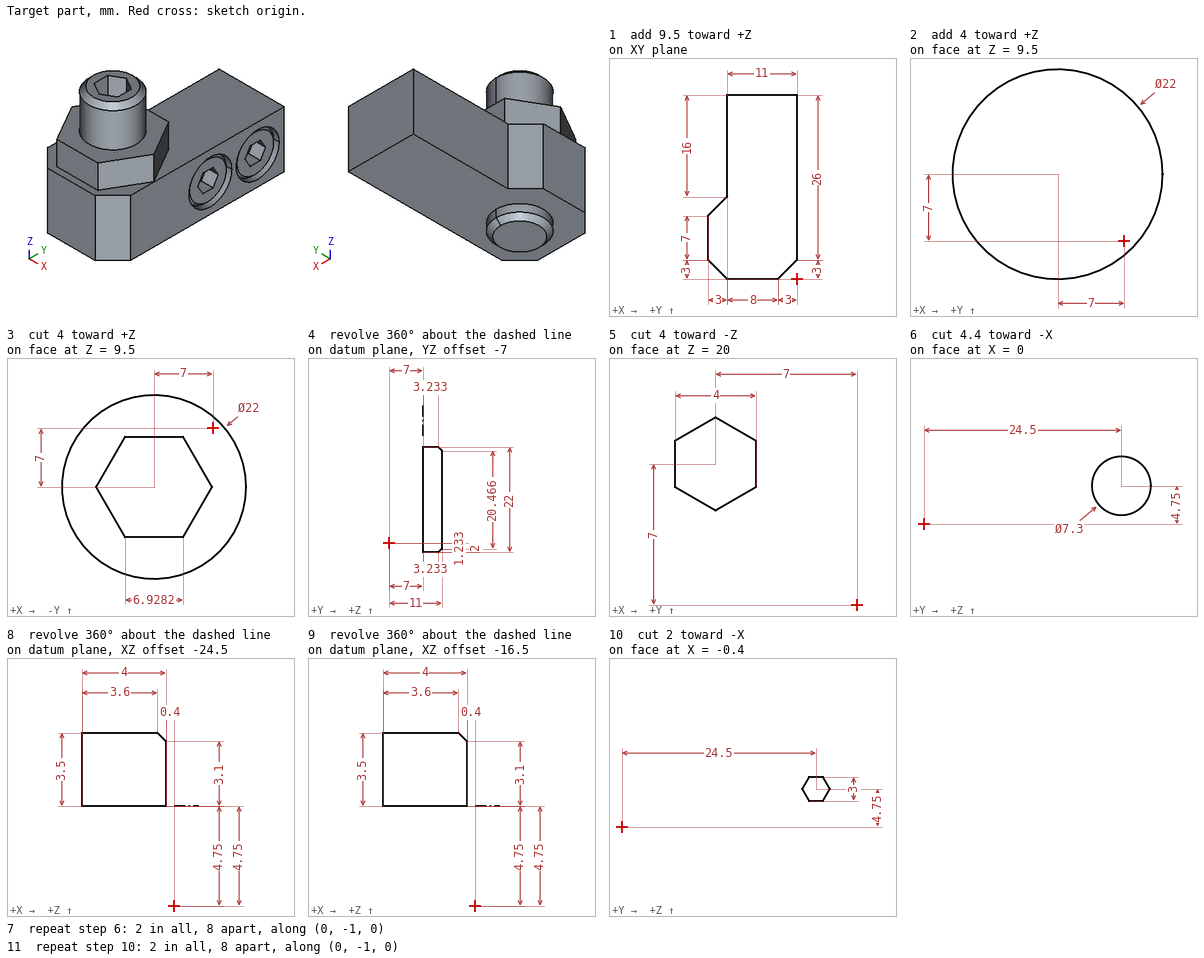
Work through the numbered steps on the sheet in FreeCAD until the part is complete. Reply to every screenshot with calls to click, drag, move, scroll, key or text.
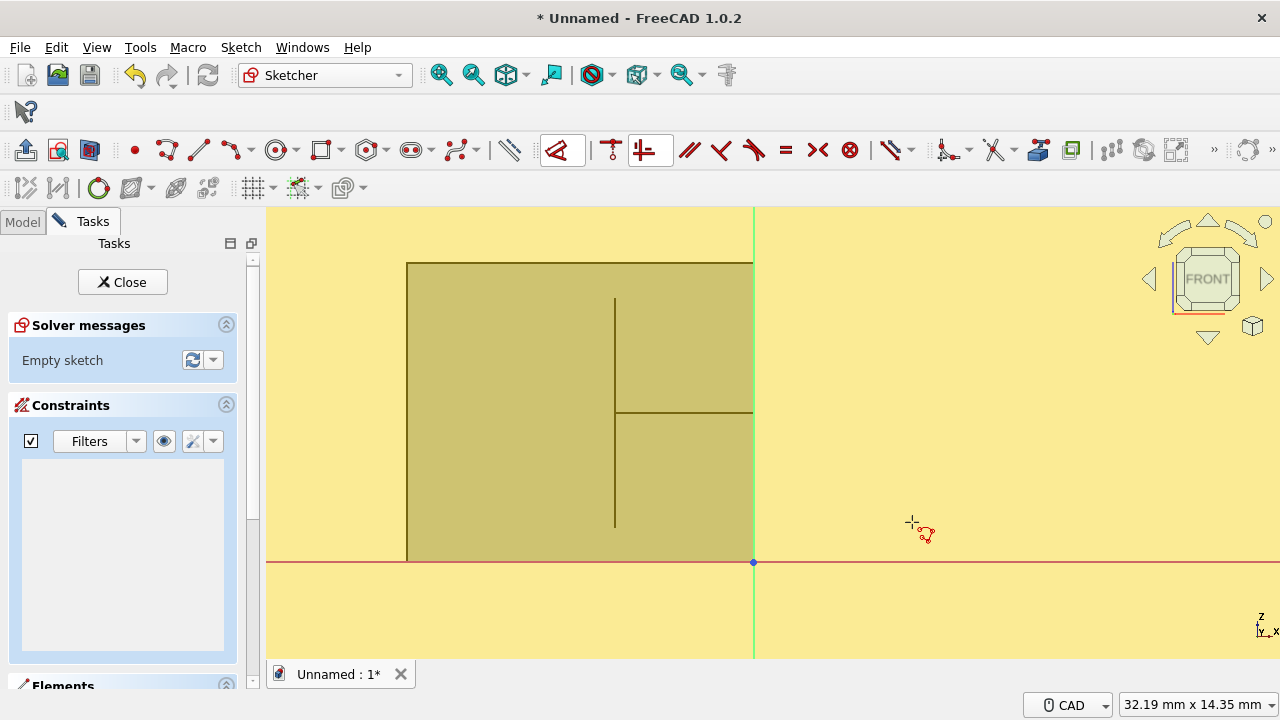
scroll(741, 413, up, 2)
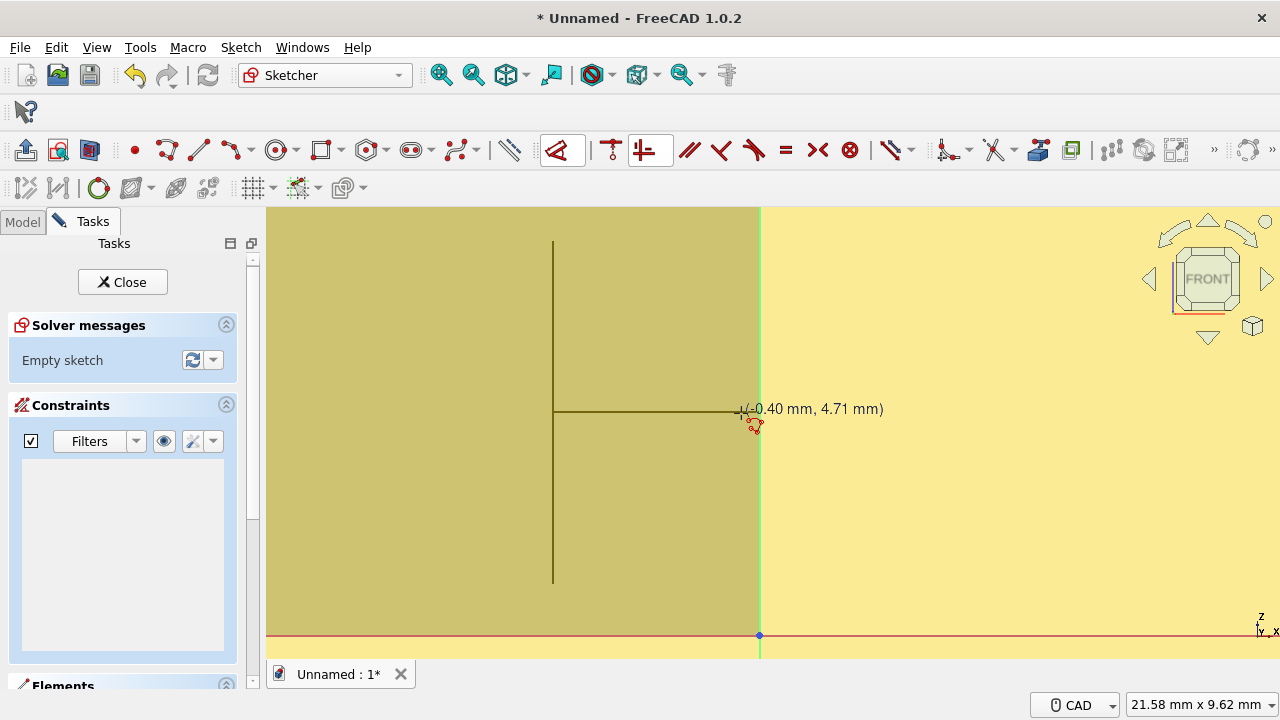
click(741, 412)
click(553, 412)
click(553, 248)
click(722, 248)
click(741, 267)
click(741, 413)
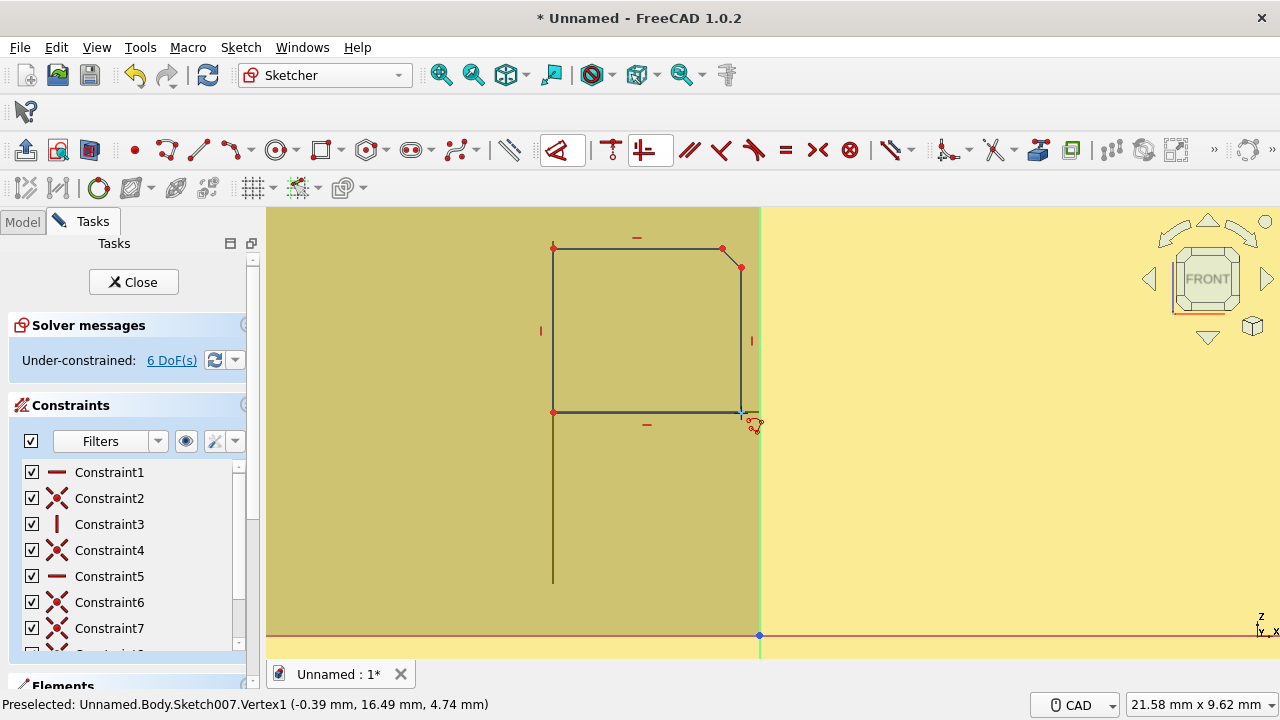
click(200, 150)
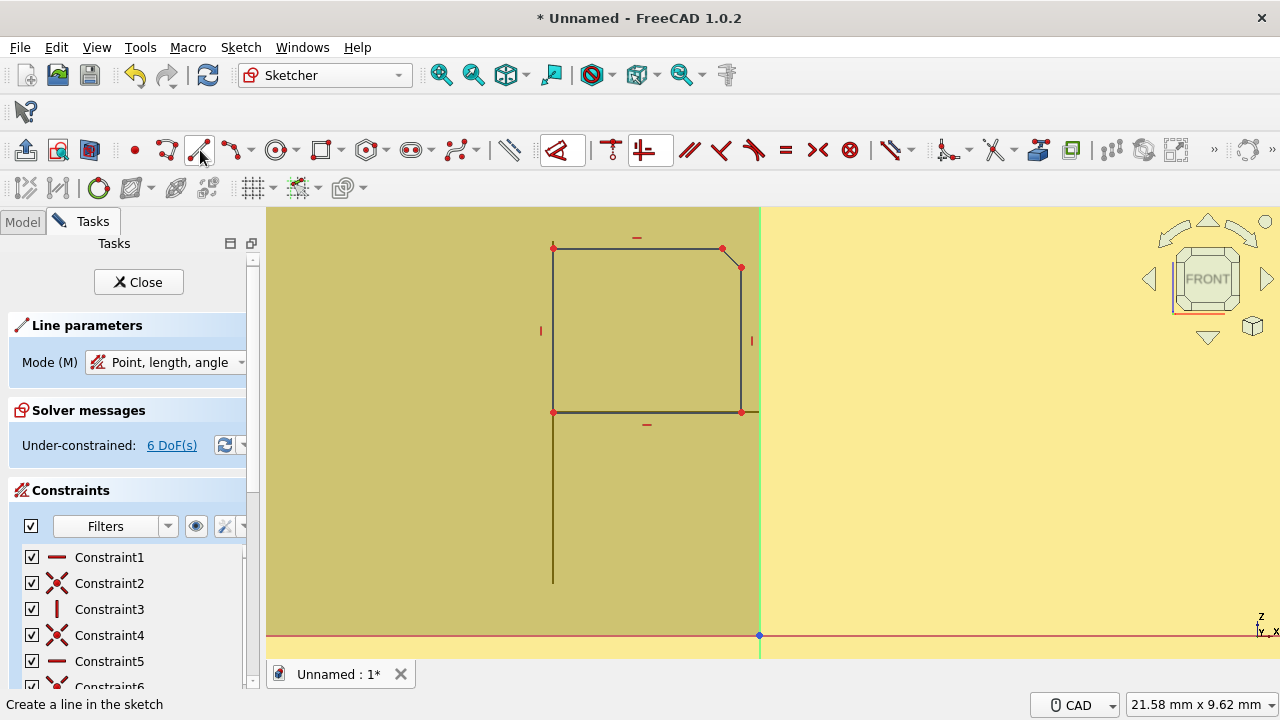
click(760, 412)
click(816, 412)
key(Escape)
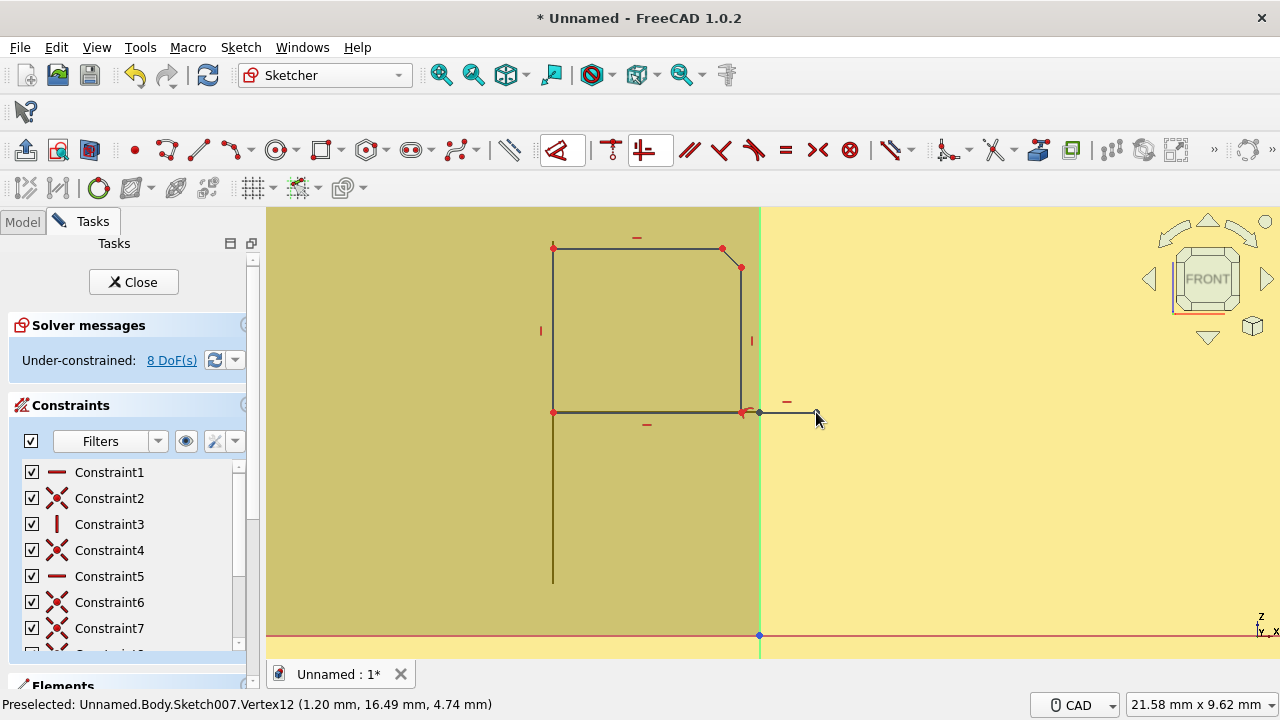
click(776, 413)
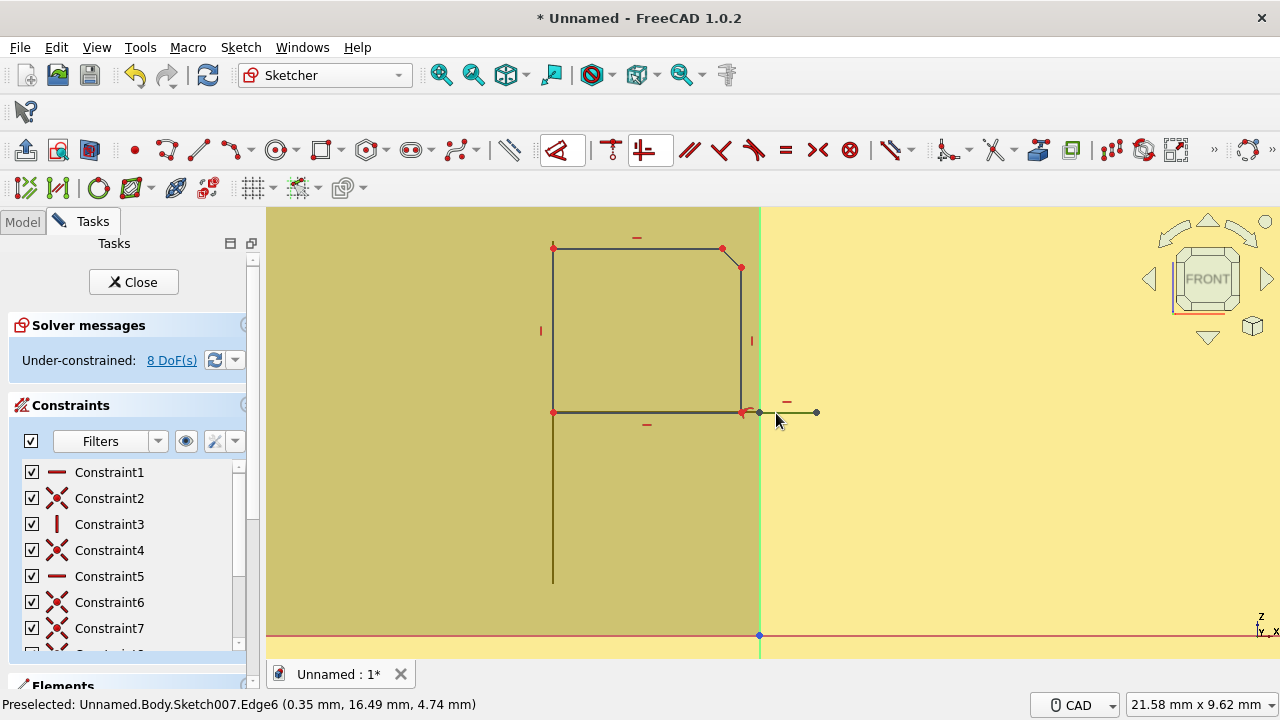
key(g)
key(n)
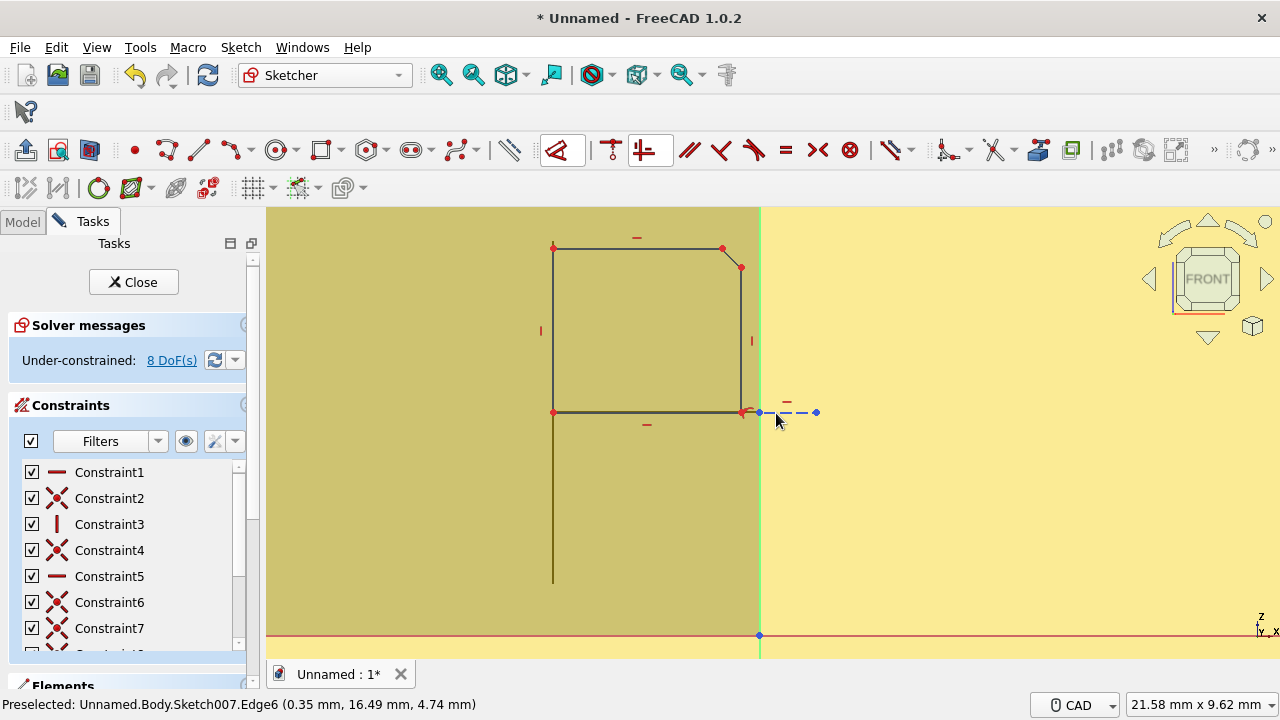
click(685, 413)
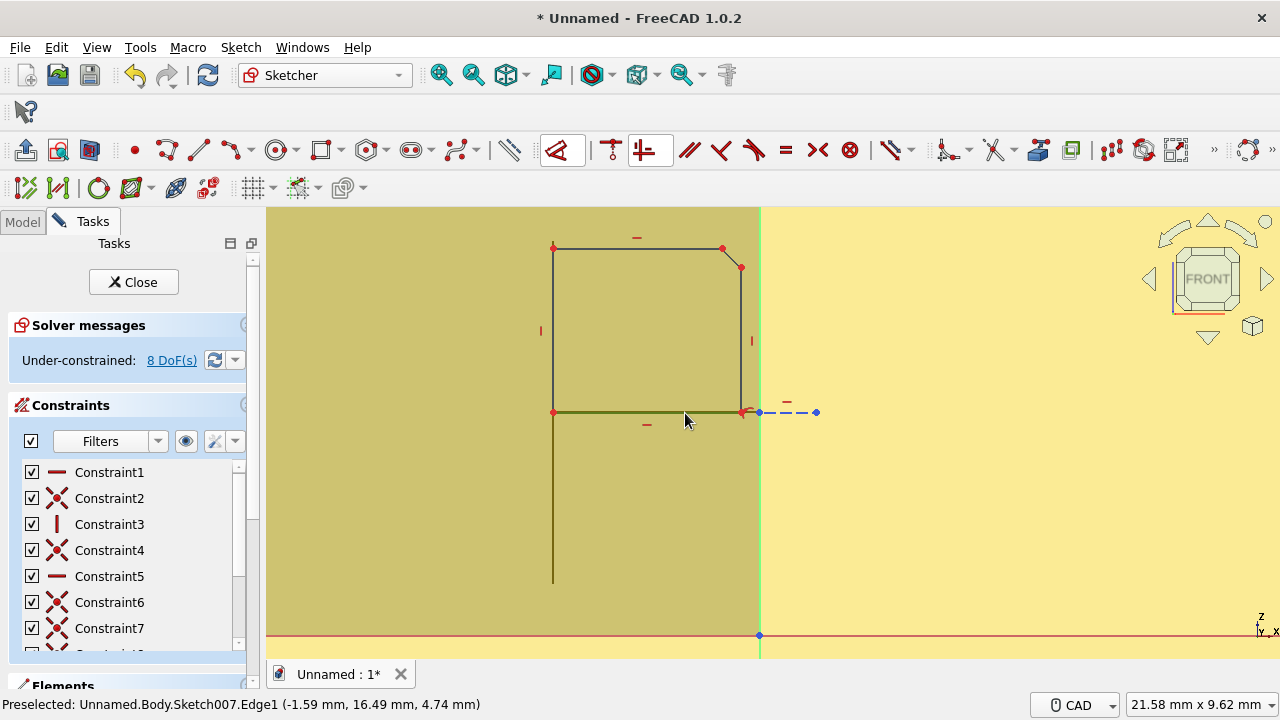
key(l)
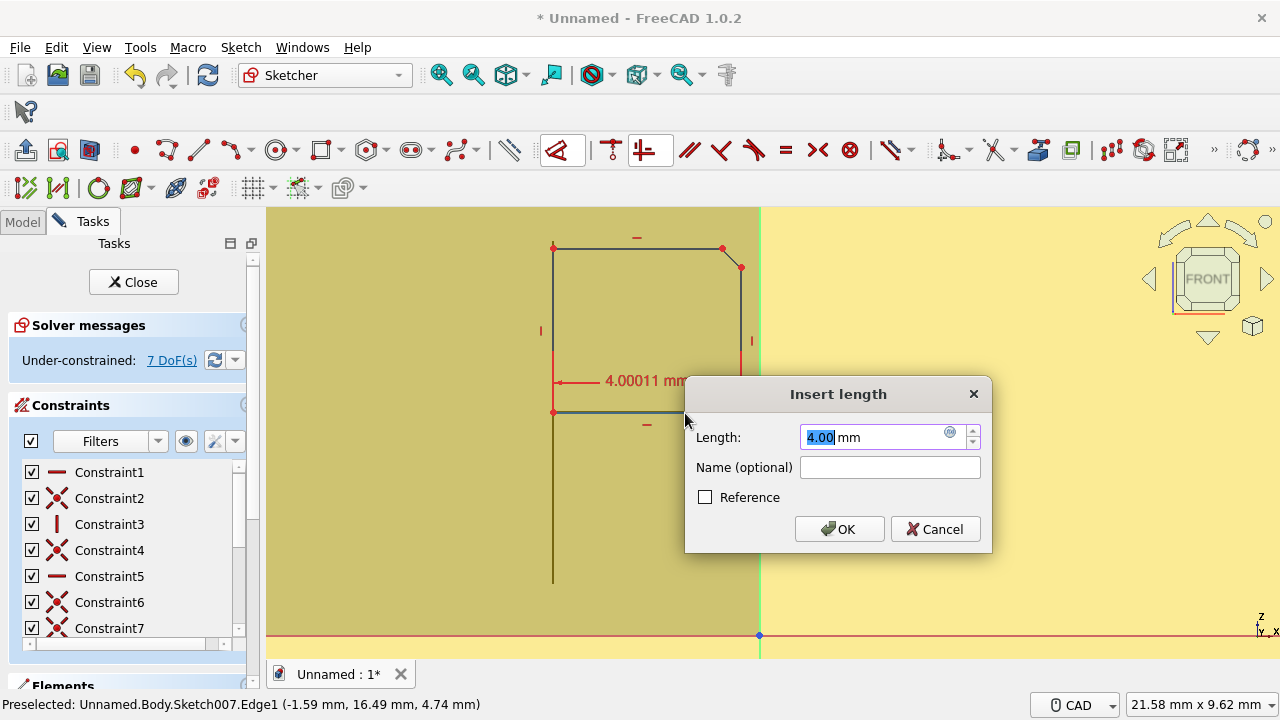
text(4)
key(Return)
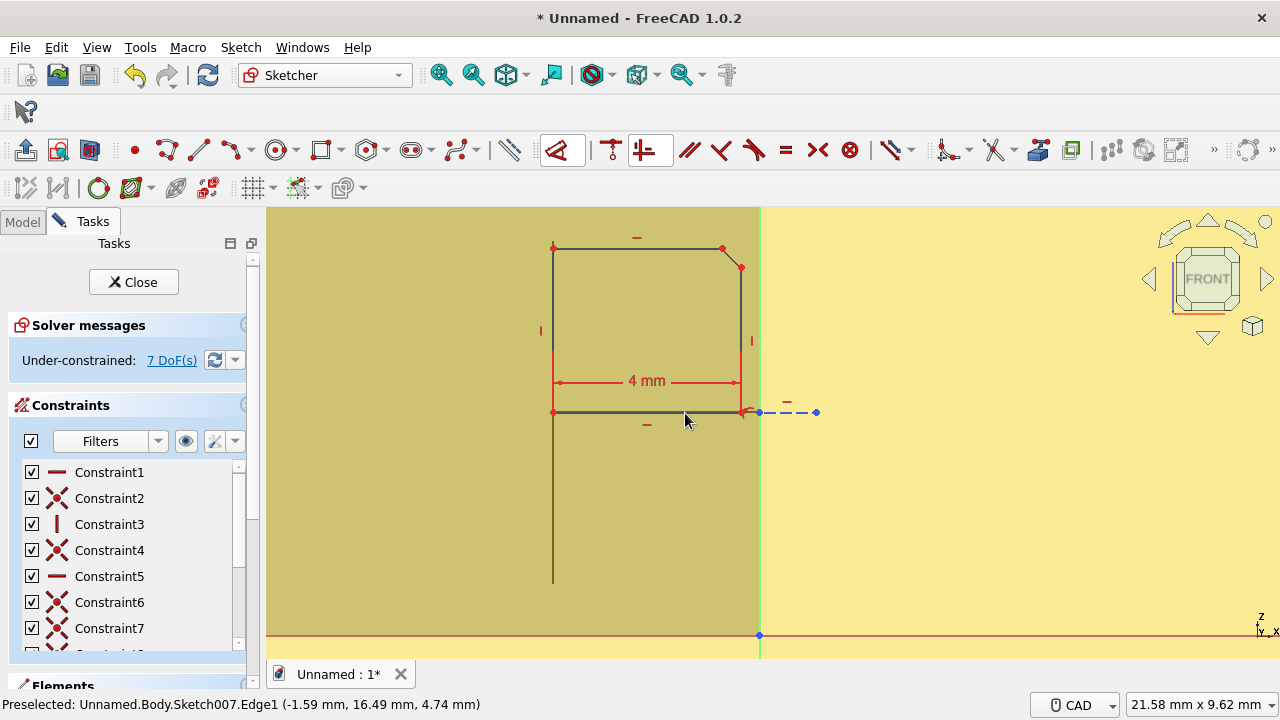
click(553, 364)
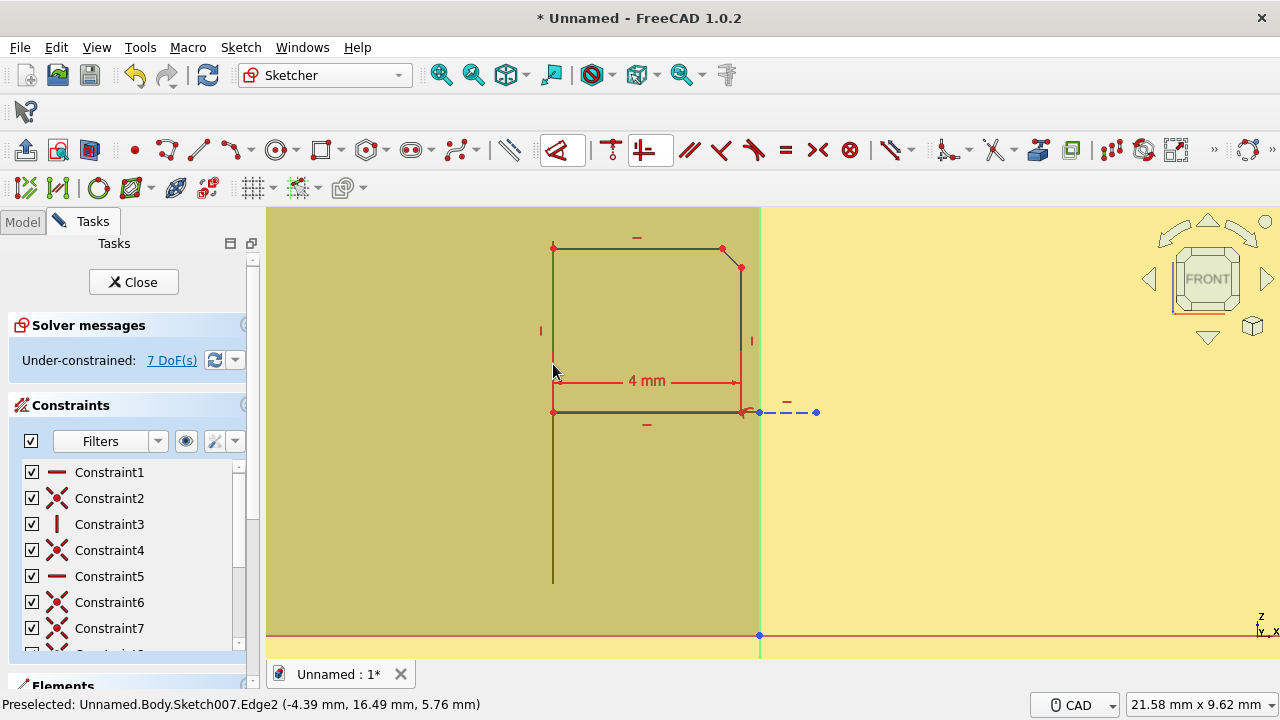
key(i)